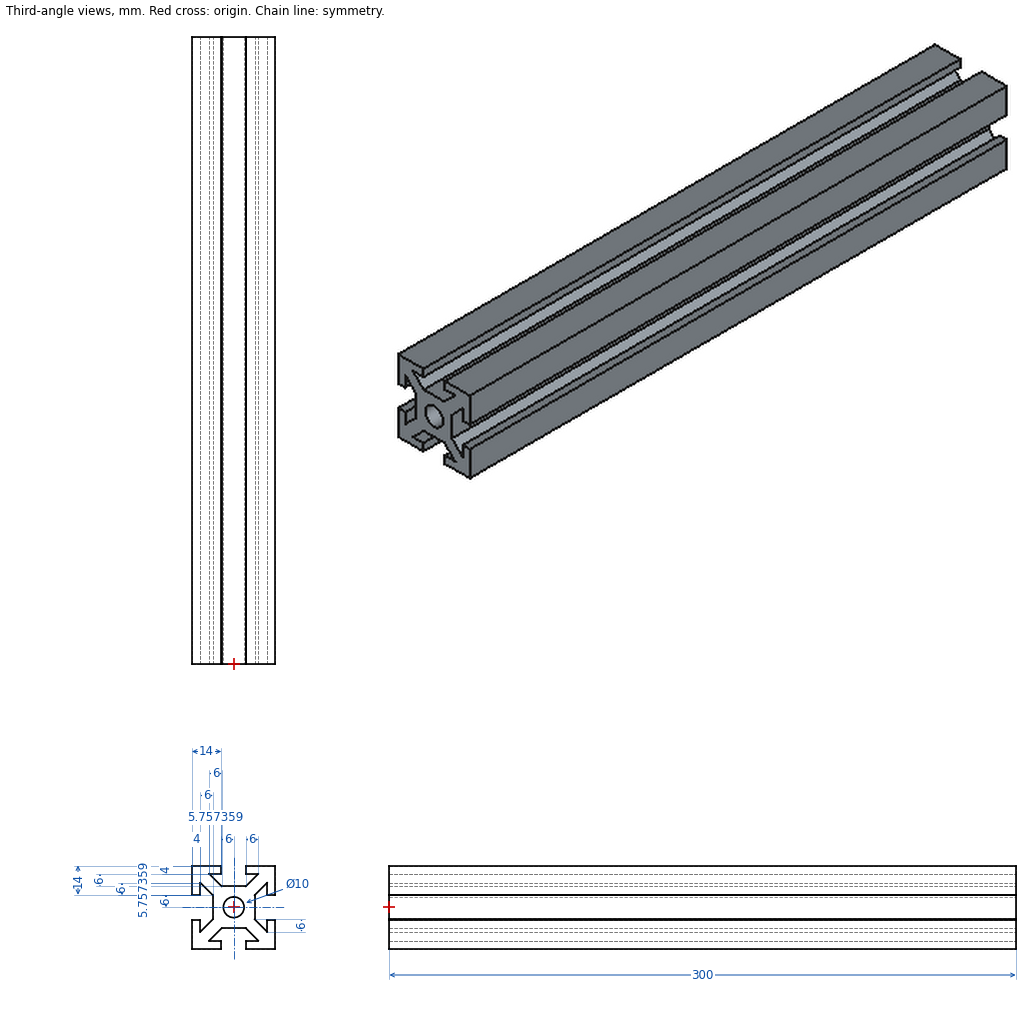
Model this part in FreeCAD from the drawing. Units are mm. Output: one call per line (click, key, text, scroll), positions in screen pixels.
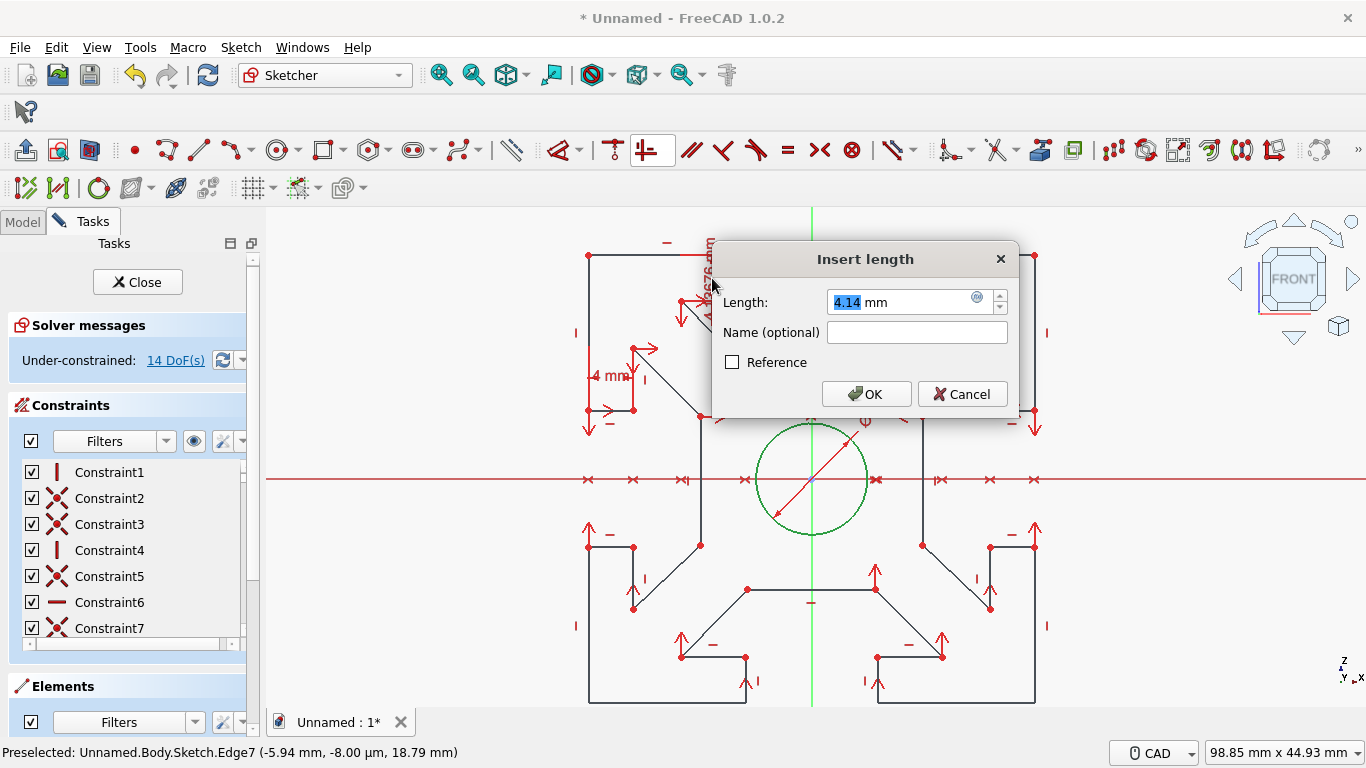
text(4)
key(Return)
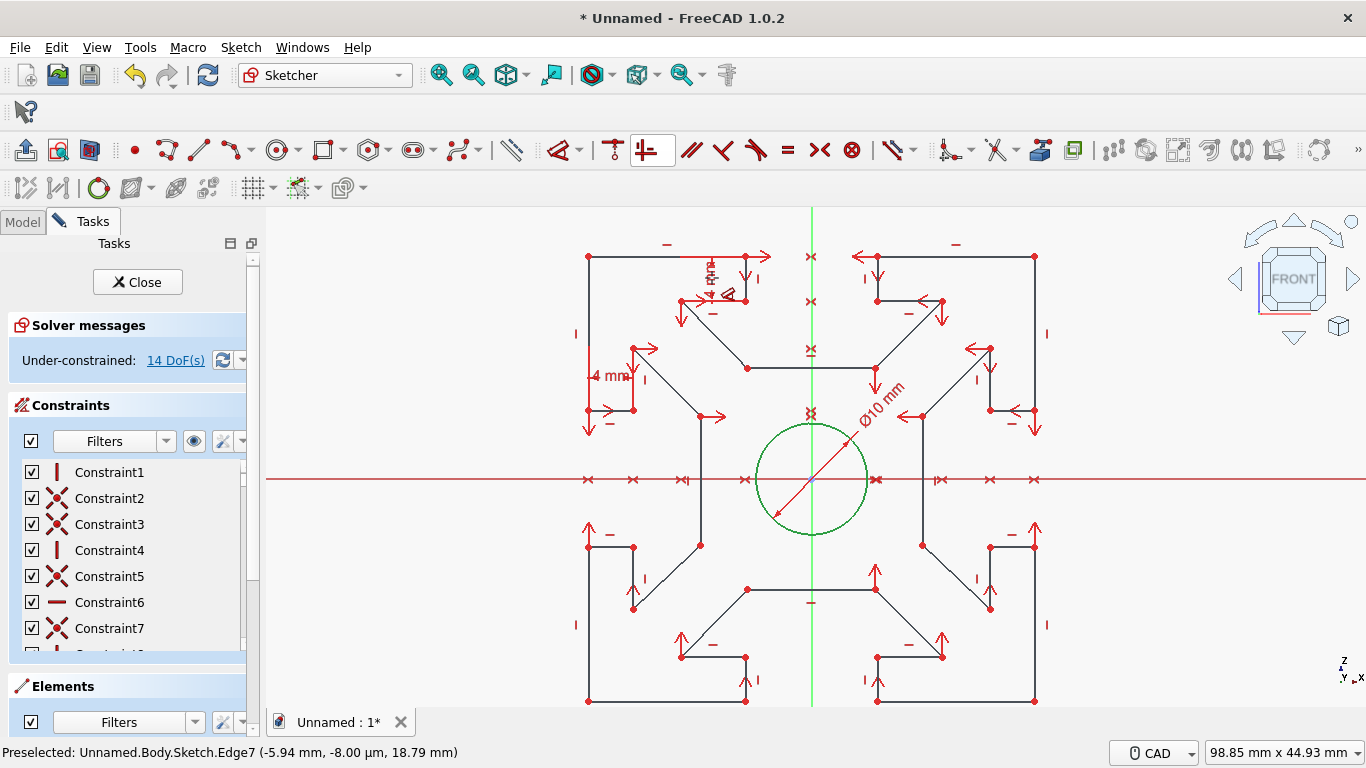
click(589, 365)
click(555, 334)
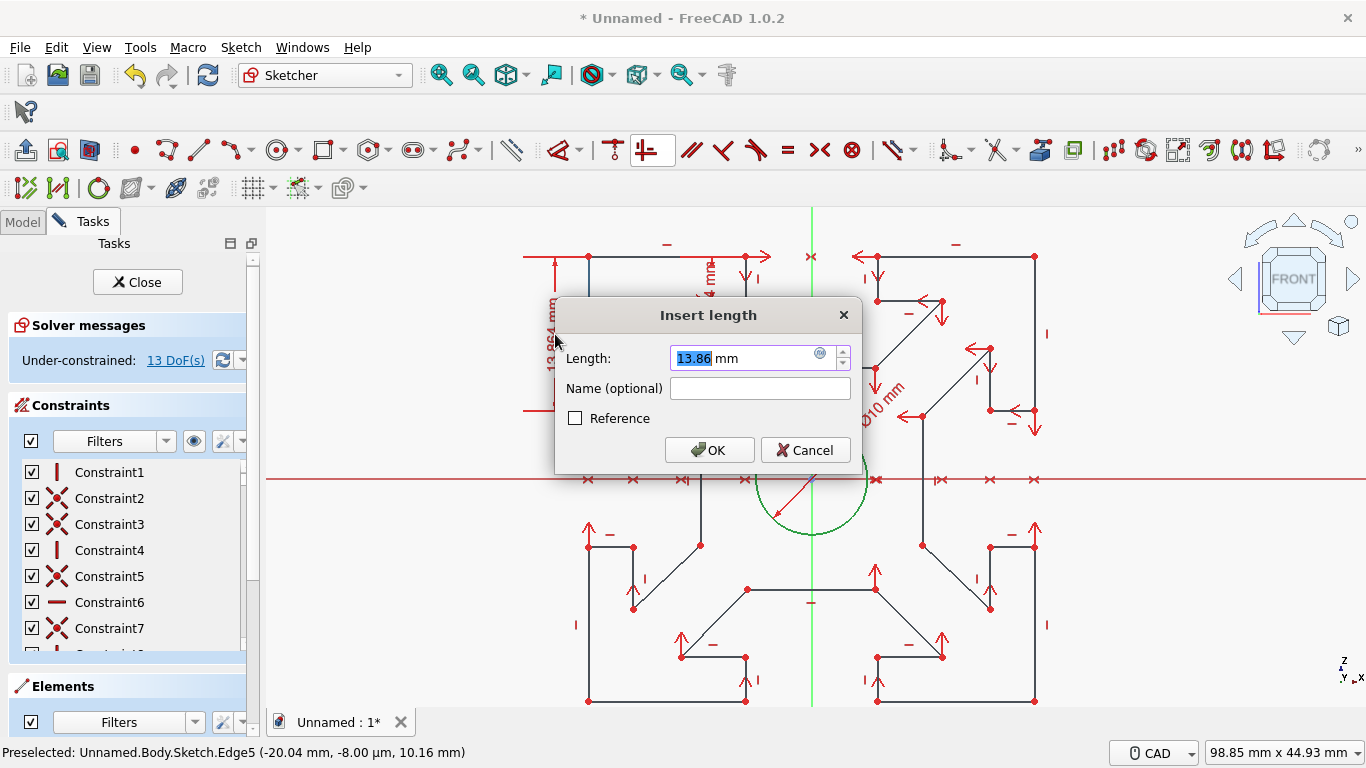
text(14)
key(Return)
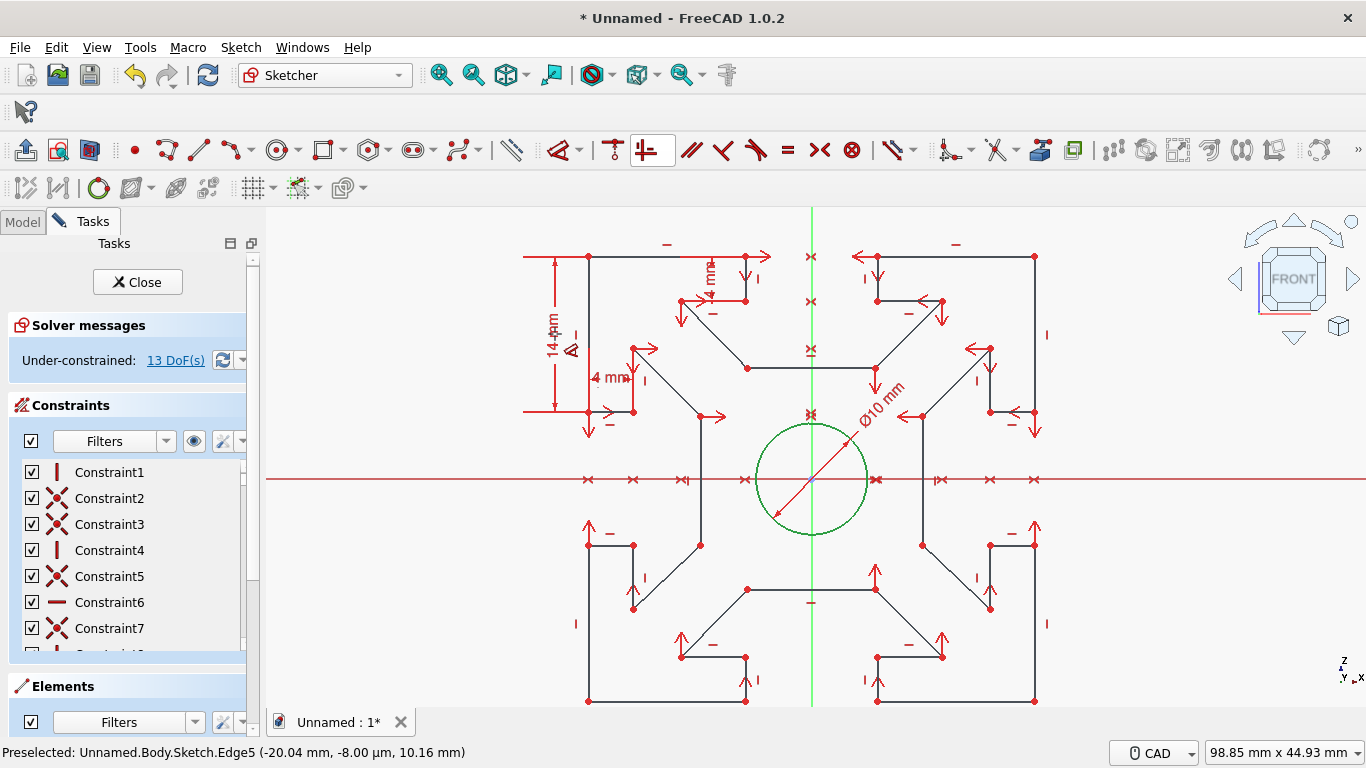
click(636, 257)
click(631, 291)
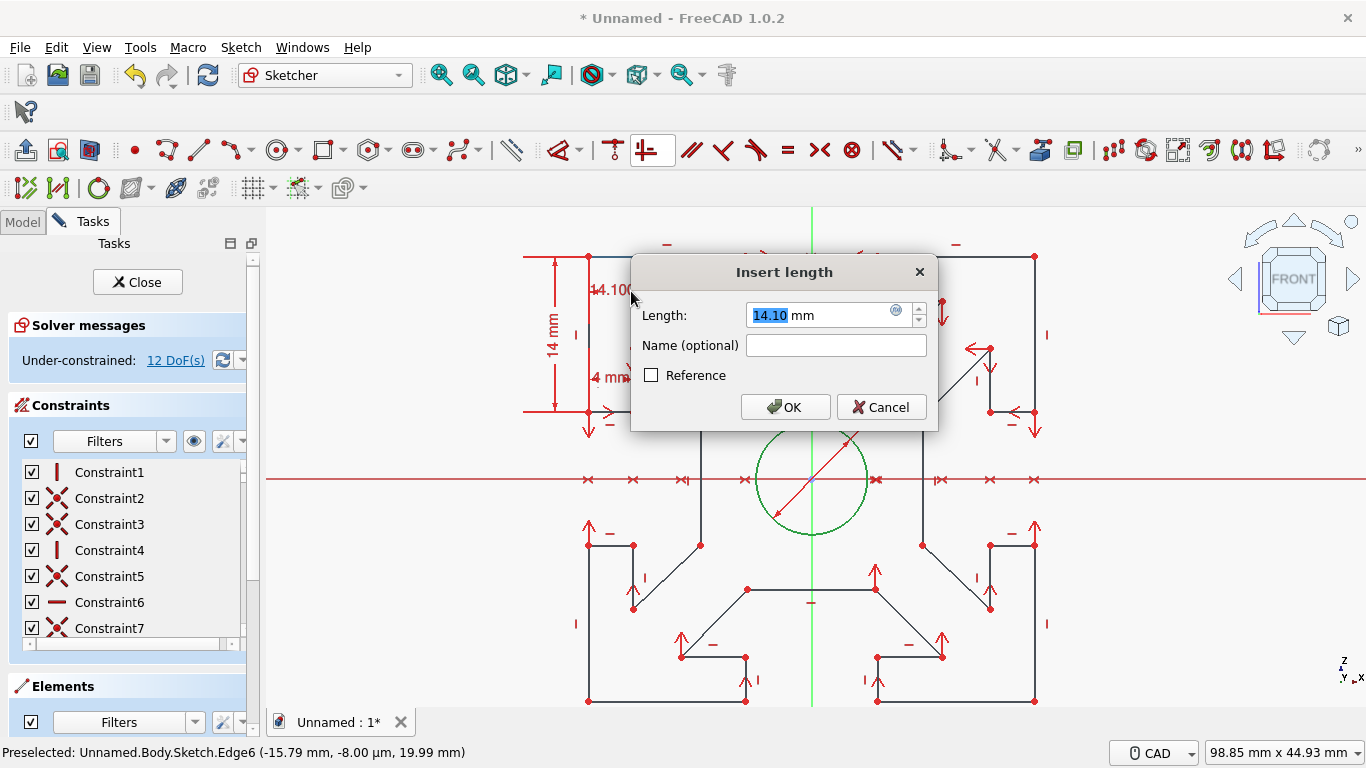
text(14)
key(Return)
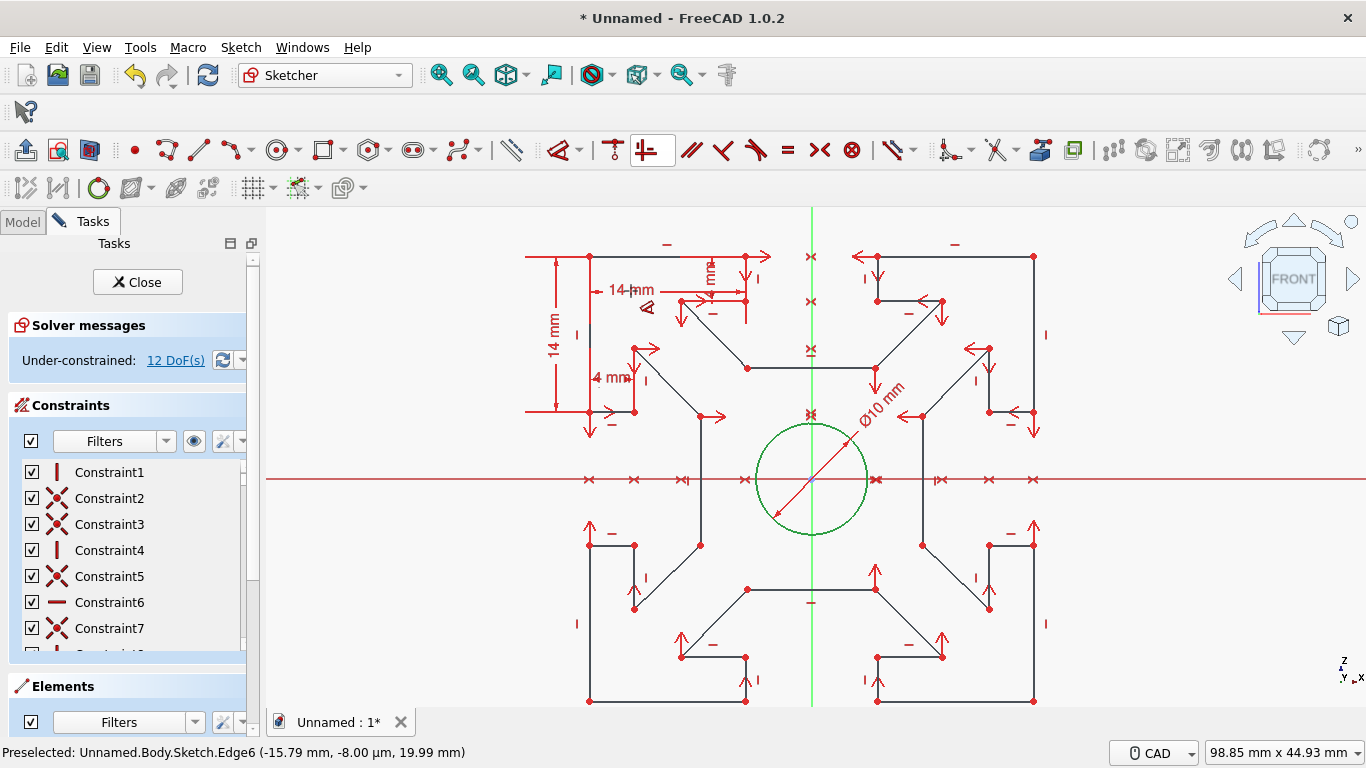
click(634, 412)
click(600, 446)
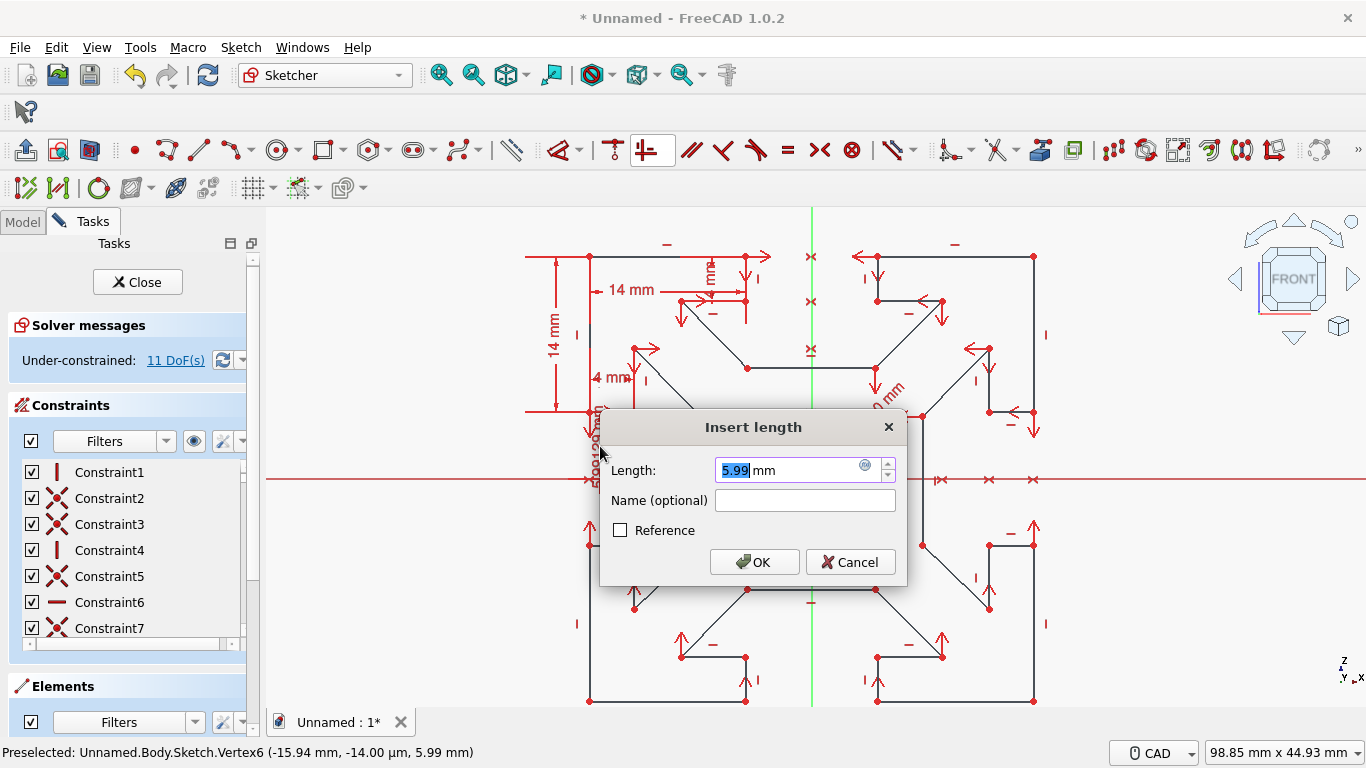
text(6)
key(Return)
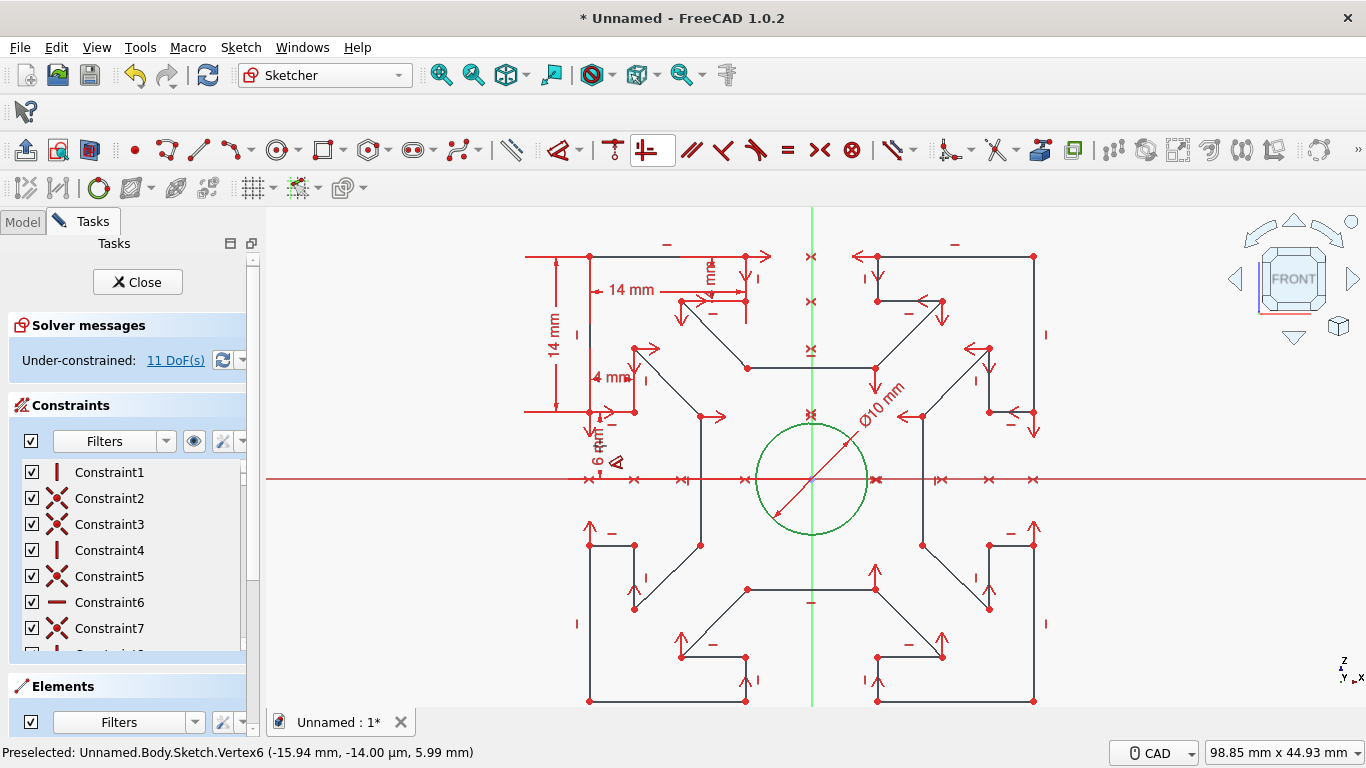
click(746, 257)
click(794, 513)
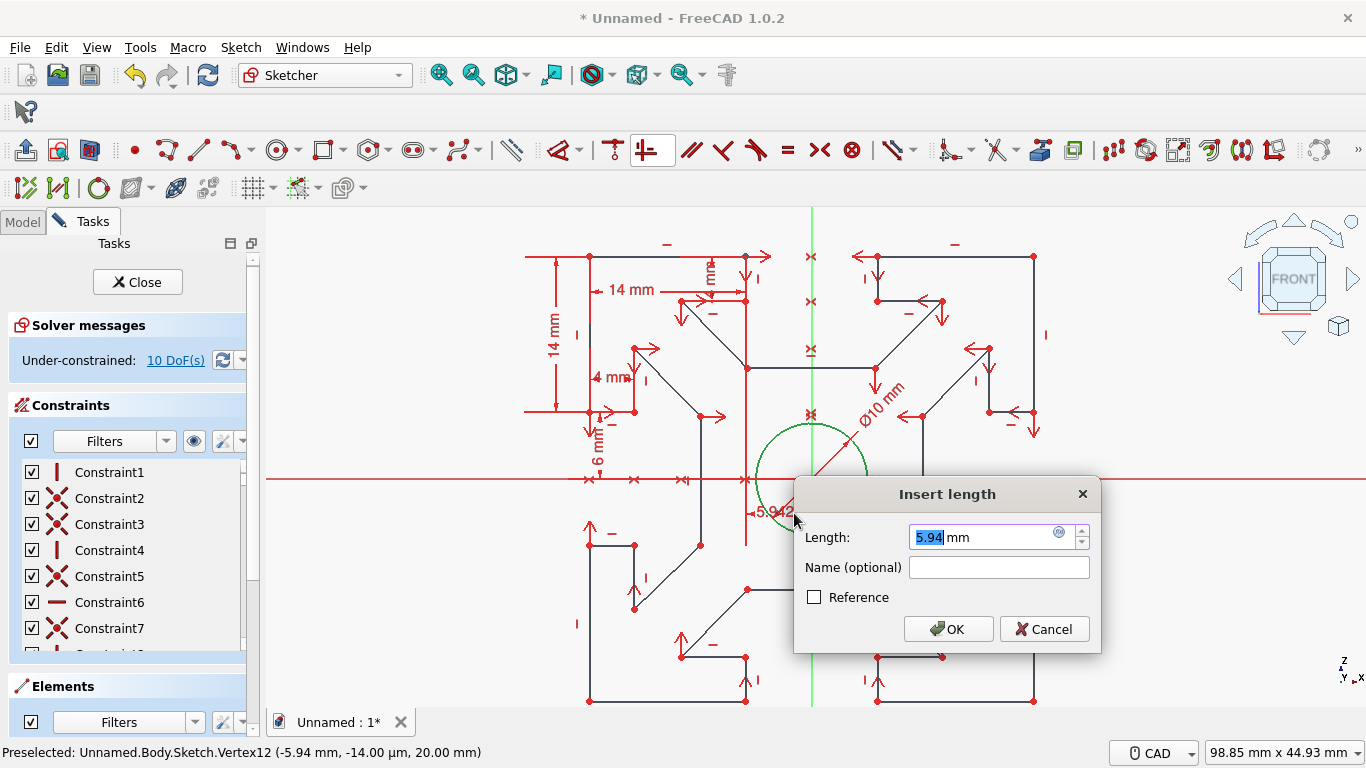
text(6)
key(Return)